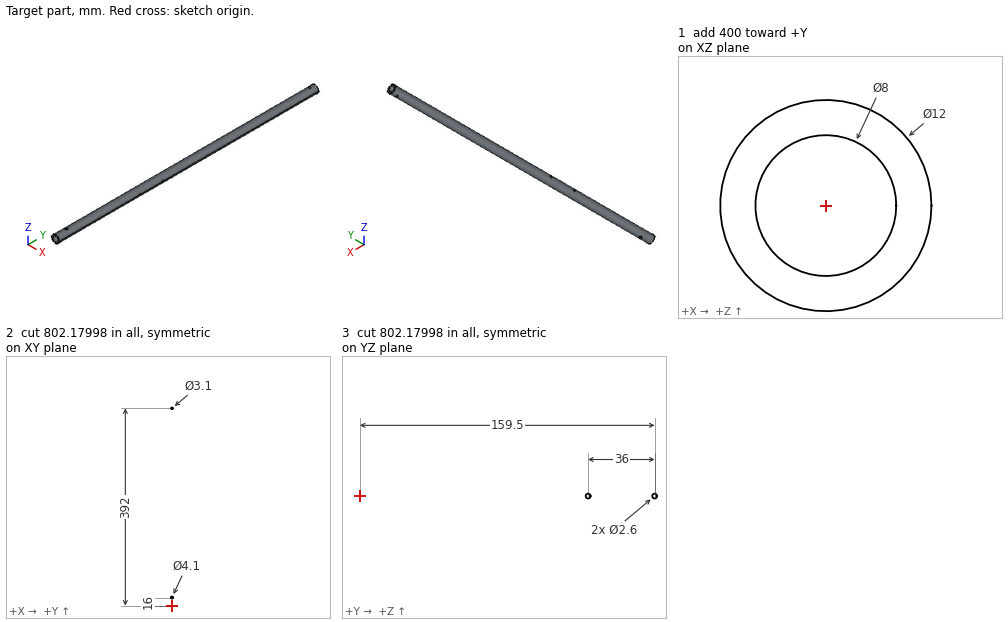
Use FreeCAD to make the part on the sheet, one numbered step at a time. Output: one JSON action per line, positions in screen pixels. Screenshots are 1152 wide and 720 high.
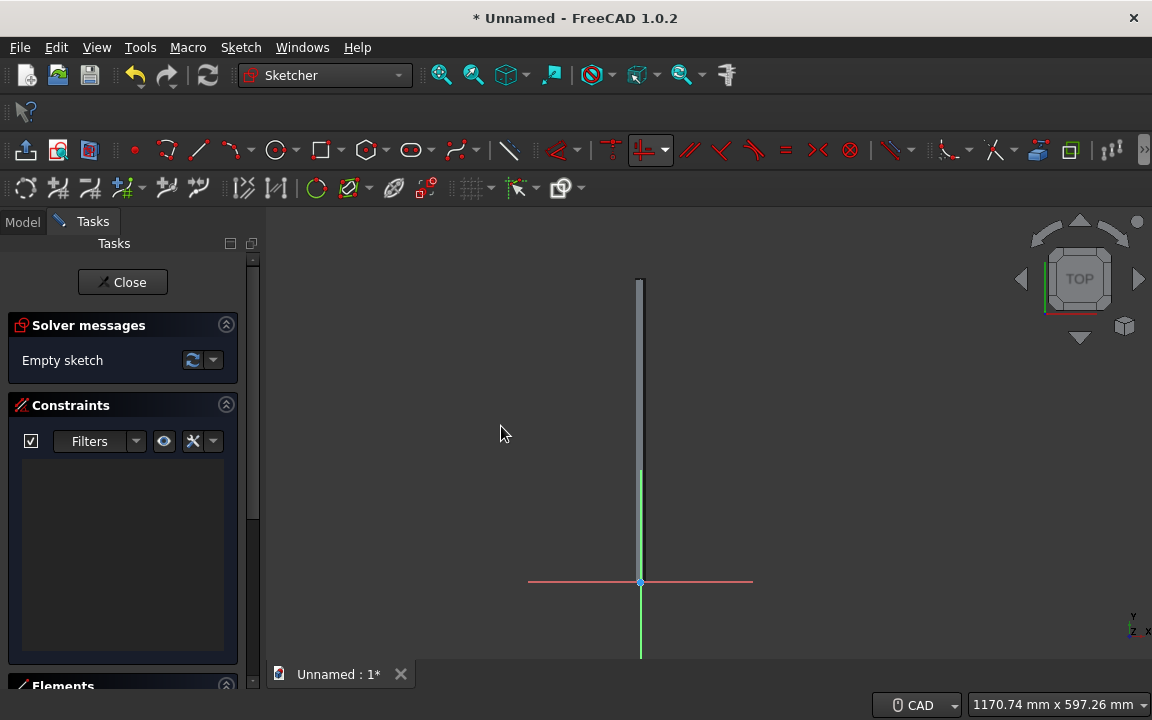
{"action": "key", "text": "g c"}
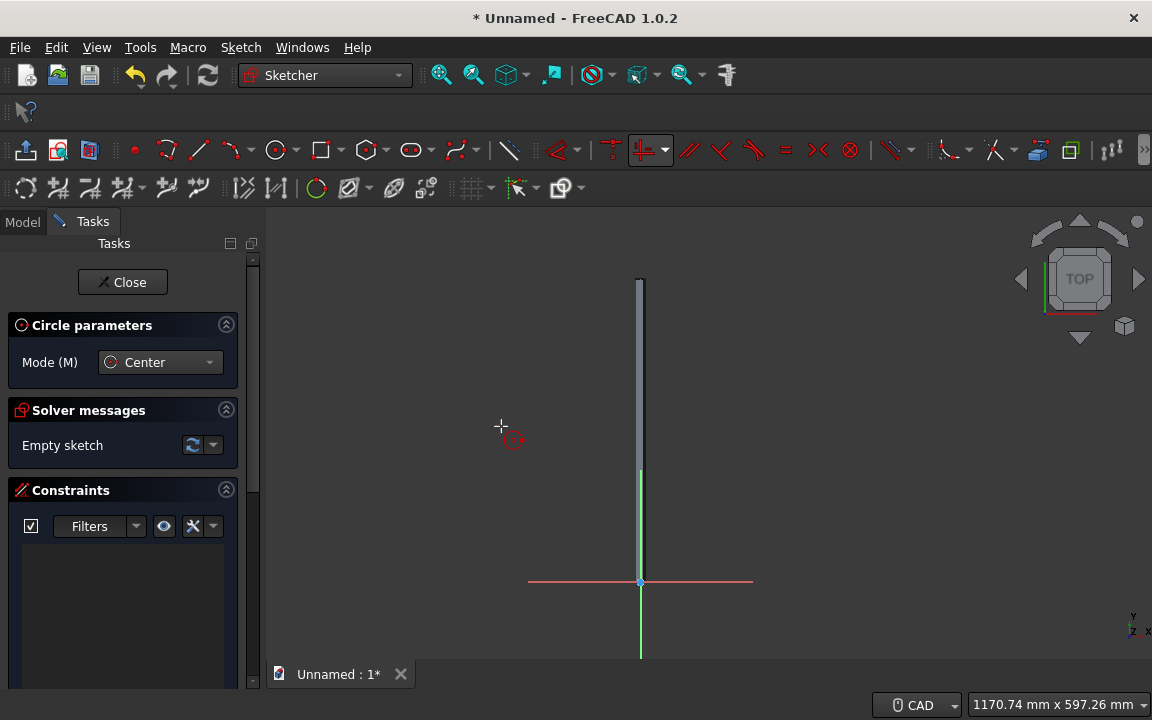
{"action": "scroll", "coordinate": [641, 570], "scroll_direction": "up", "scroll_amount": 14}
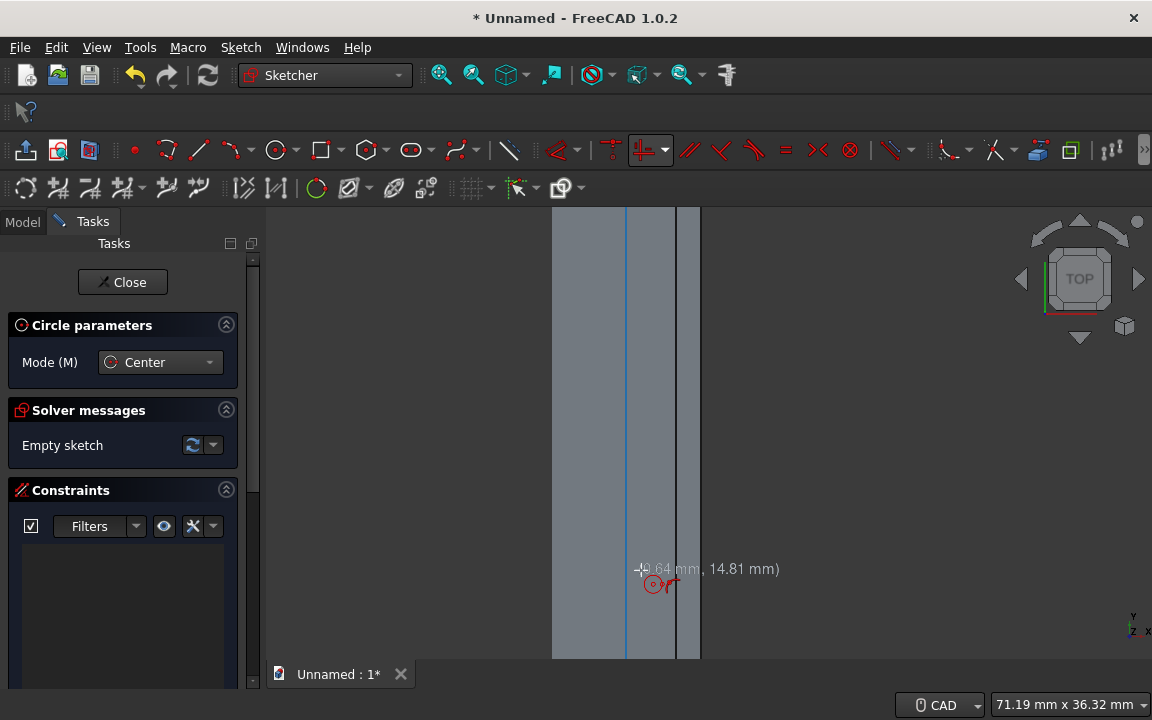
{"action": "scroll", "coordinate": [641, 570], "scroll_direction": "down", "scroll_amount": 14}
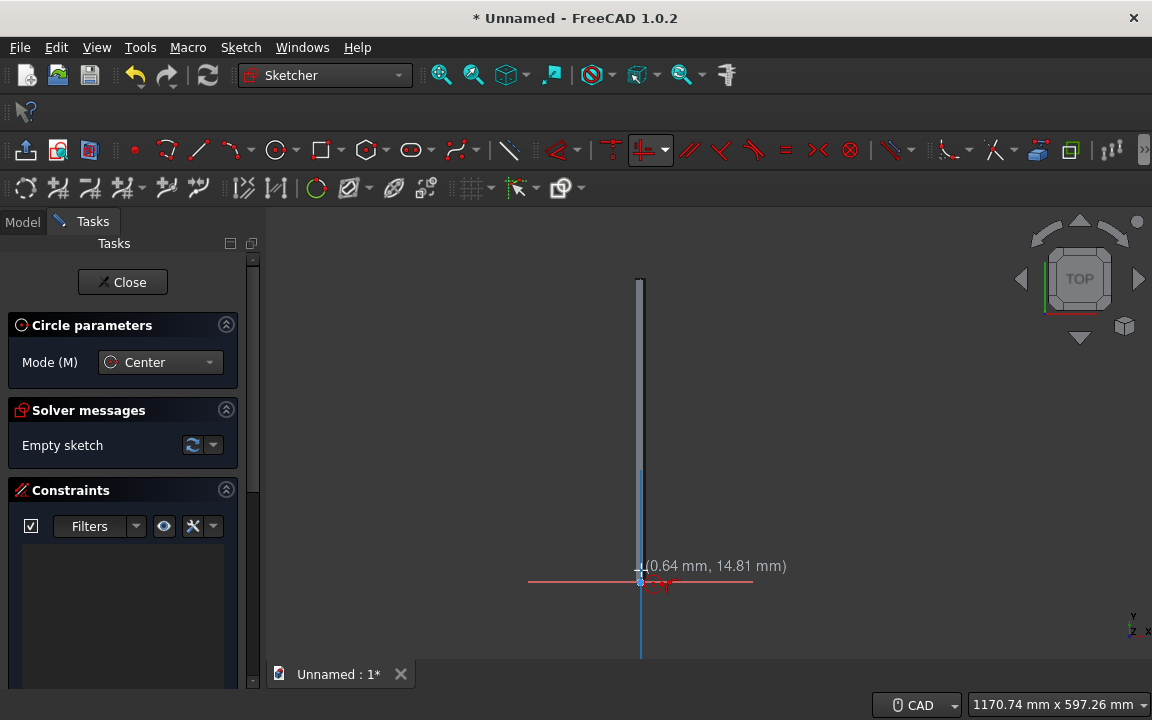
{"action": "scroll", "coordinate": [641, 570], "scroll_direction": "up", "scroll_amount": 2}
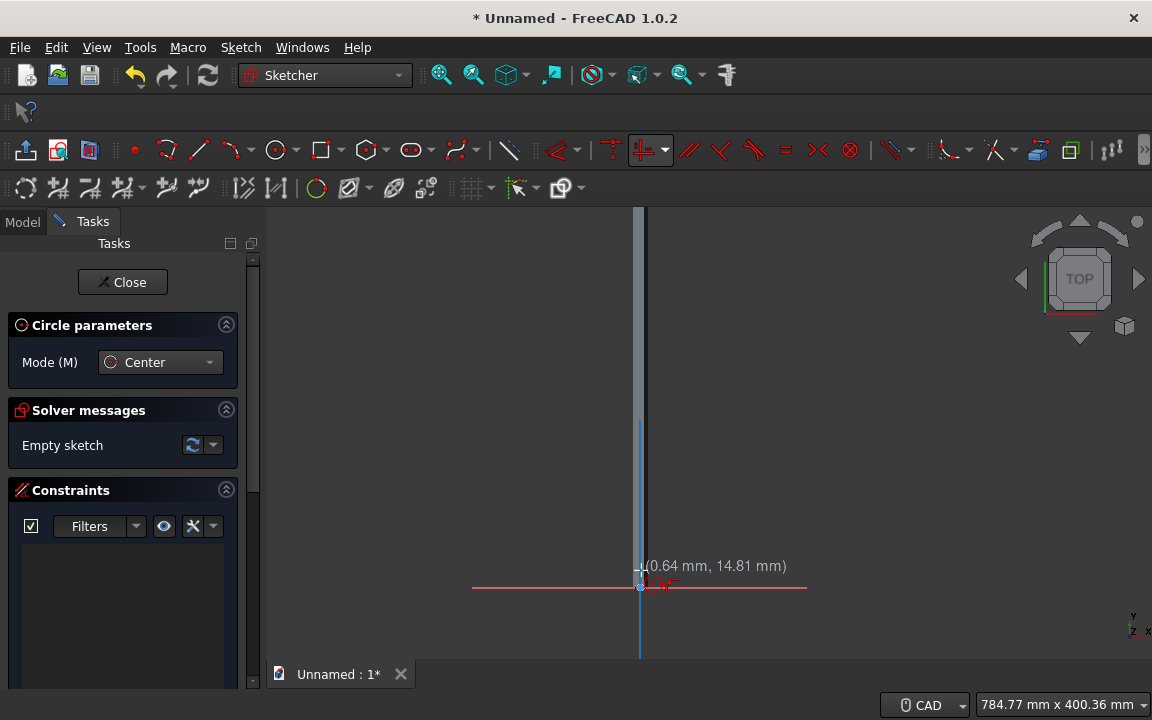
{"action": "left_click", "coordinate": [640, 570]}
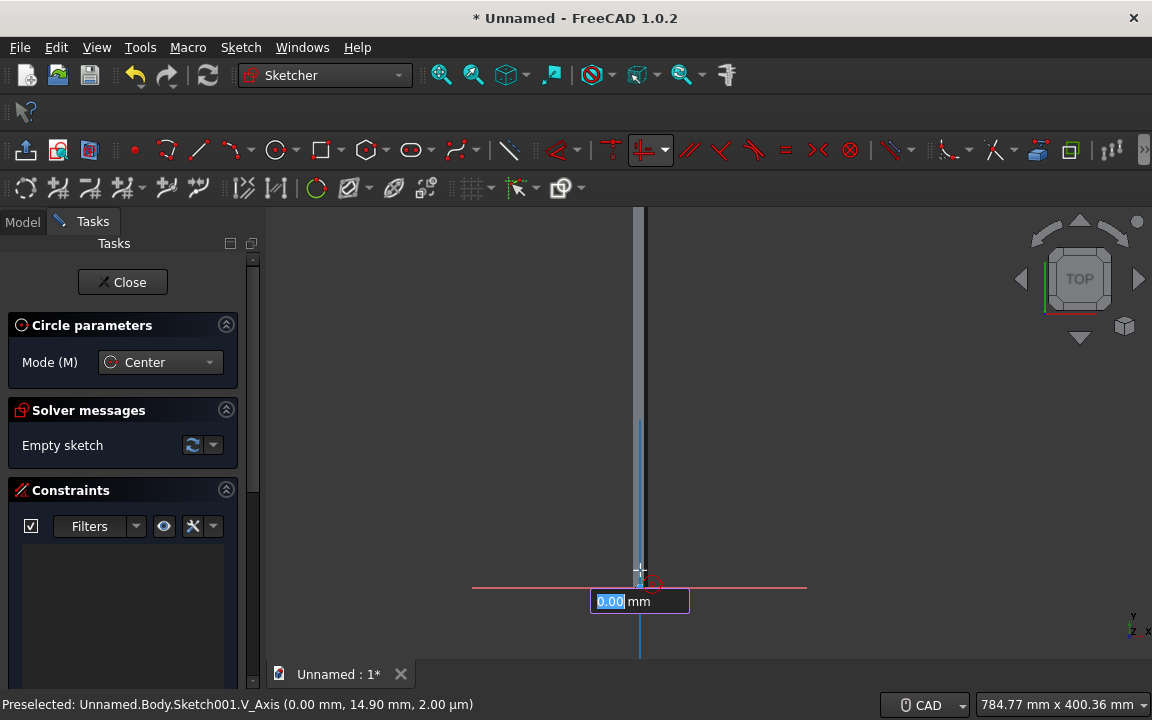
{"action": "scroll", "coordinate": [642, 569], "scroll_direction": "up", "scroll_amount": 10}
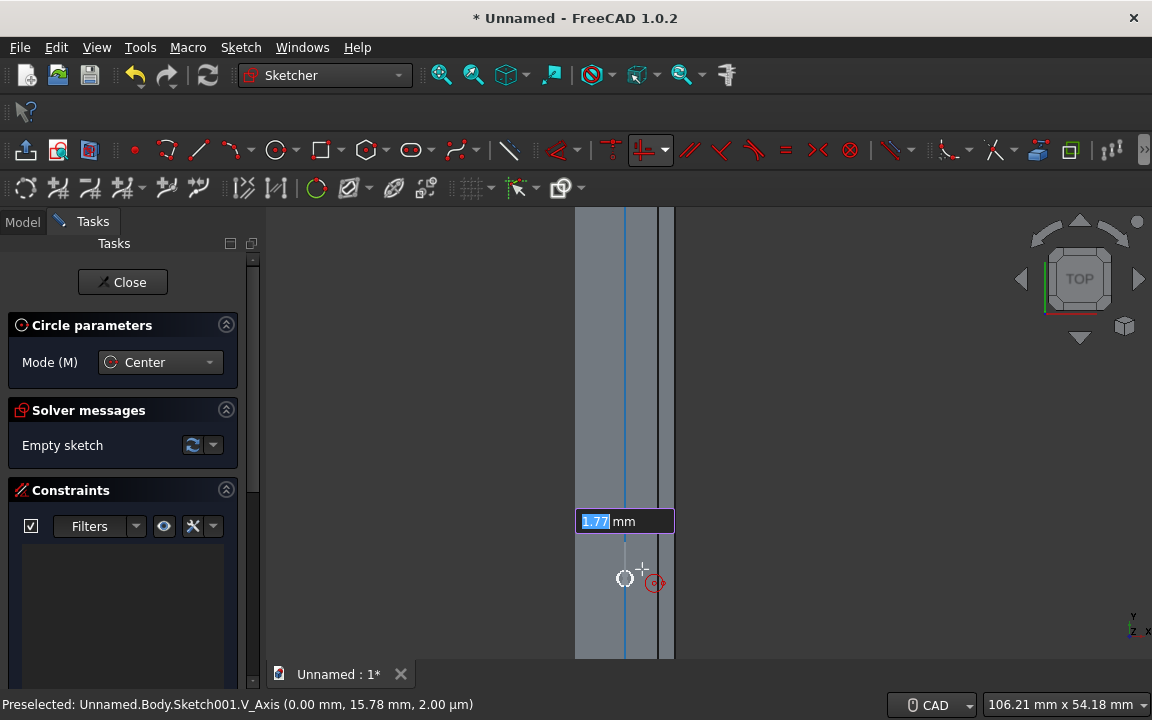
{"action": "left_click", "coordinate": [641, 564]}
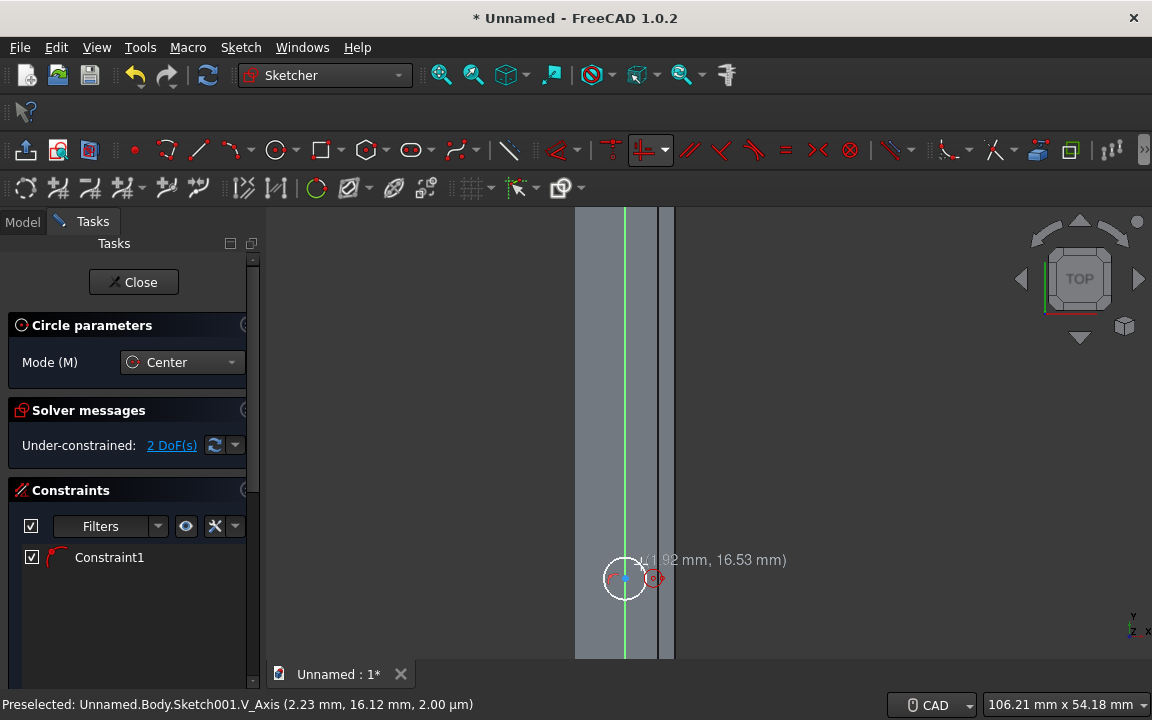
{"action": "scroll", "coordinate": [642, 570], "scroll_direction": "down", "scroll_amount": 12}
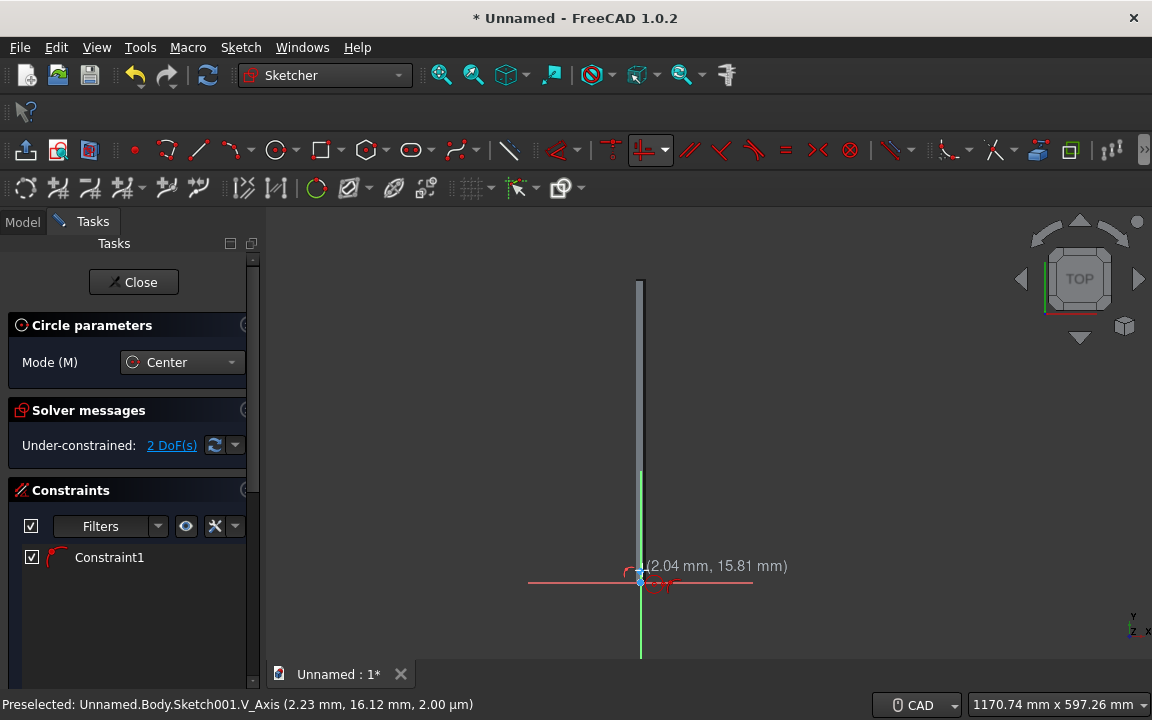
{"action": "scroll", "coordinate": [641, 286], "scroll_direction": "up", "scroll_amount": 15}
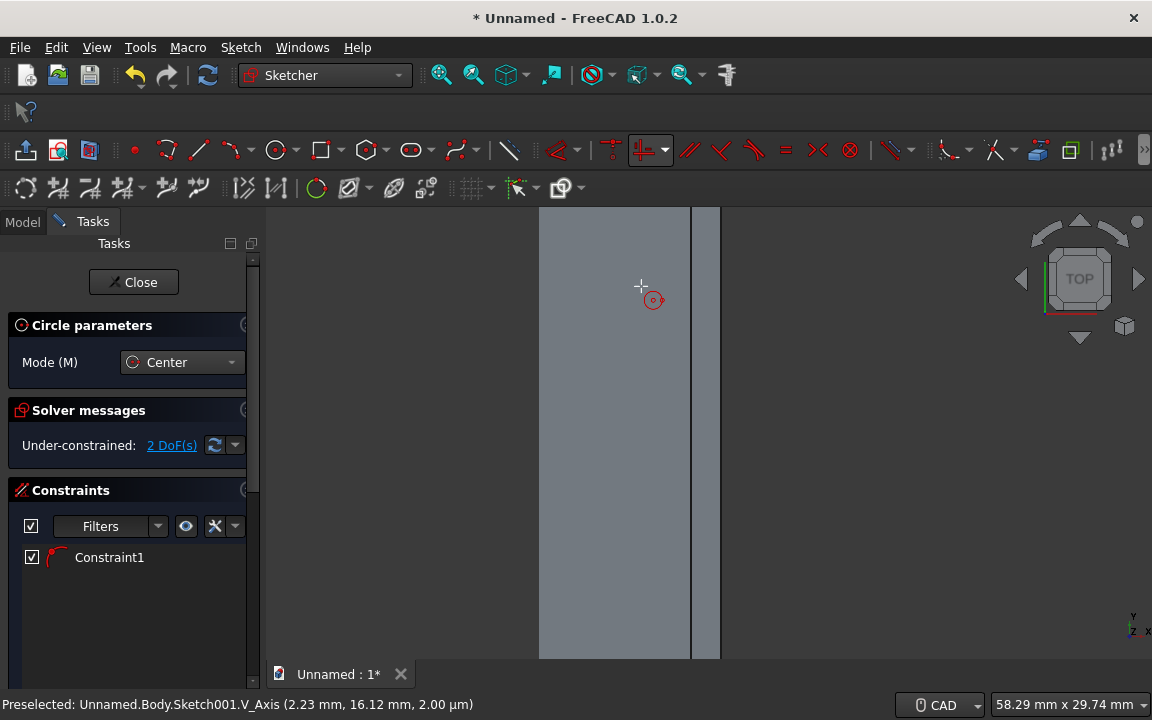
{"action": "scroll", "coordinate": [641, 285], "scroll_direction": "down", "scroll_amount": 15}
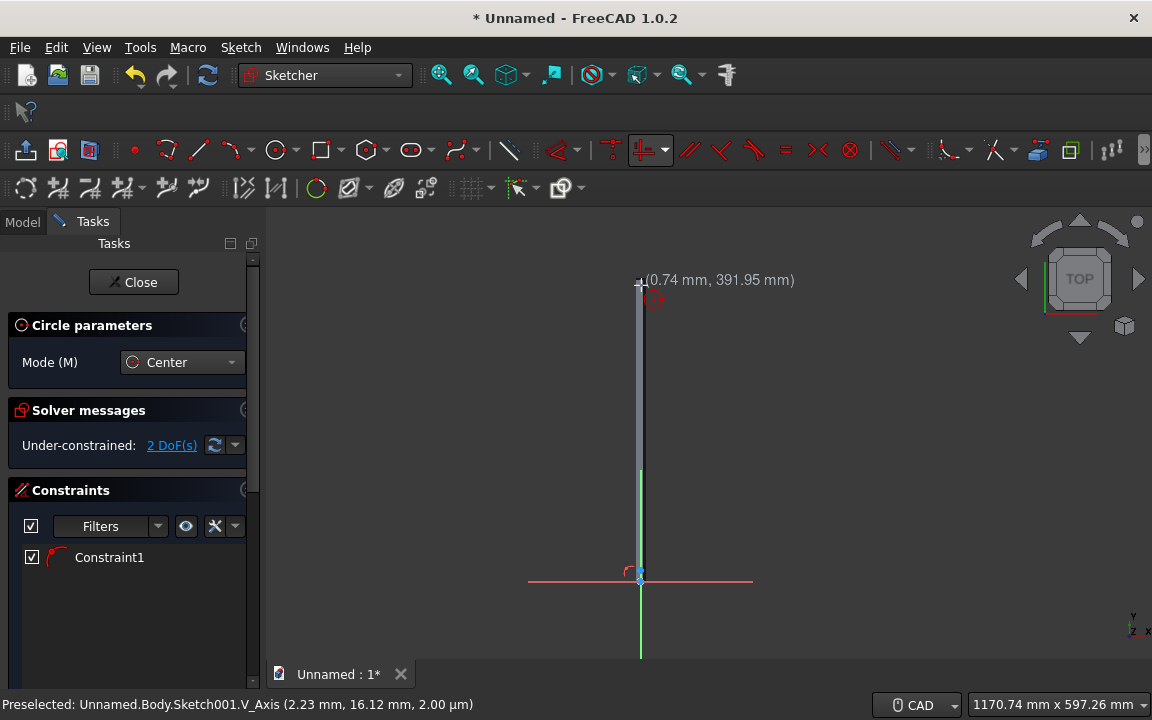
{"action": "left_click", "coordinate": [641, 285]}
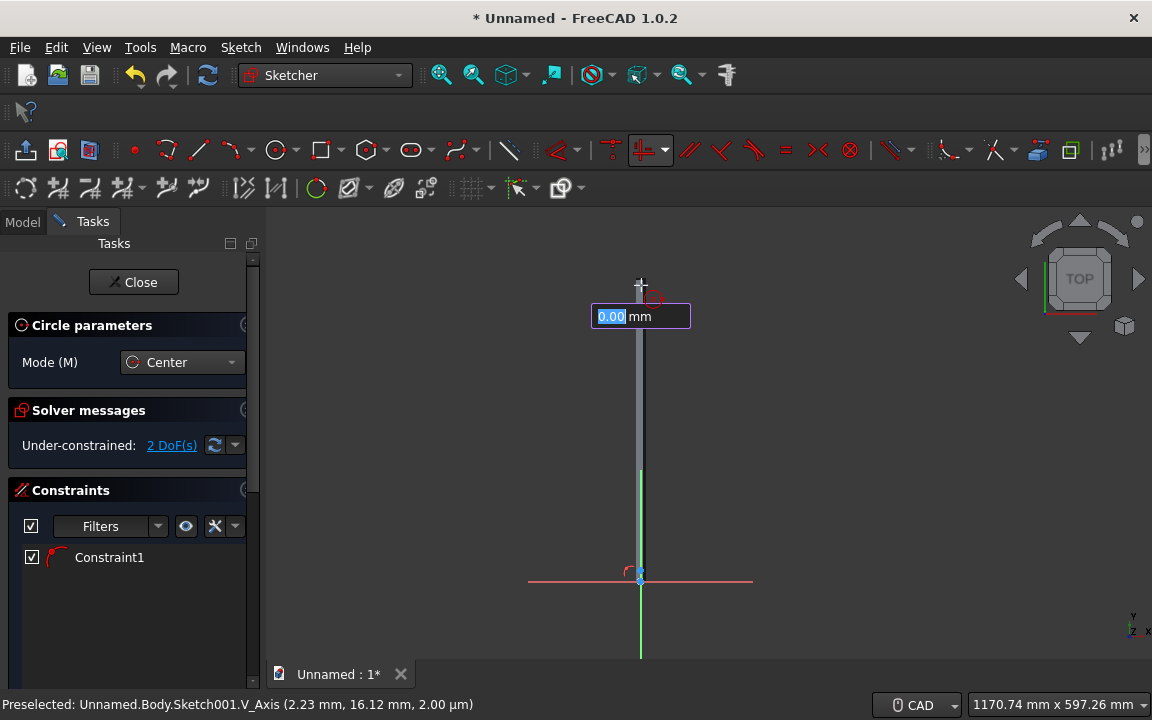
{"action": "scroll", "coordinate": [642, 285], "scroll_direction": "up", "scroll_amount": 14}